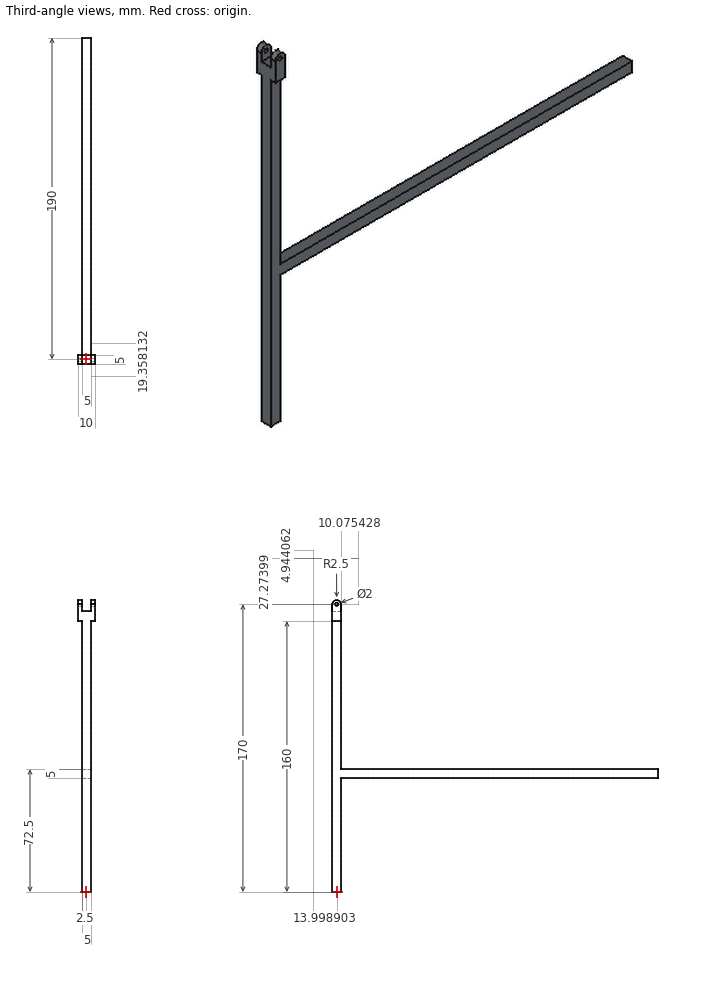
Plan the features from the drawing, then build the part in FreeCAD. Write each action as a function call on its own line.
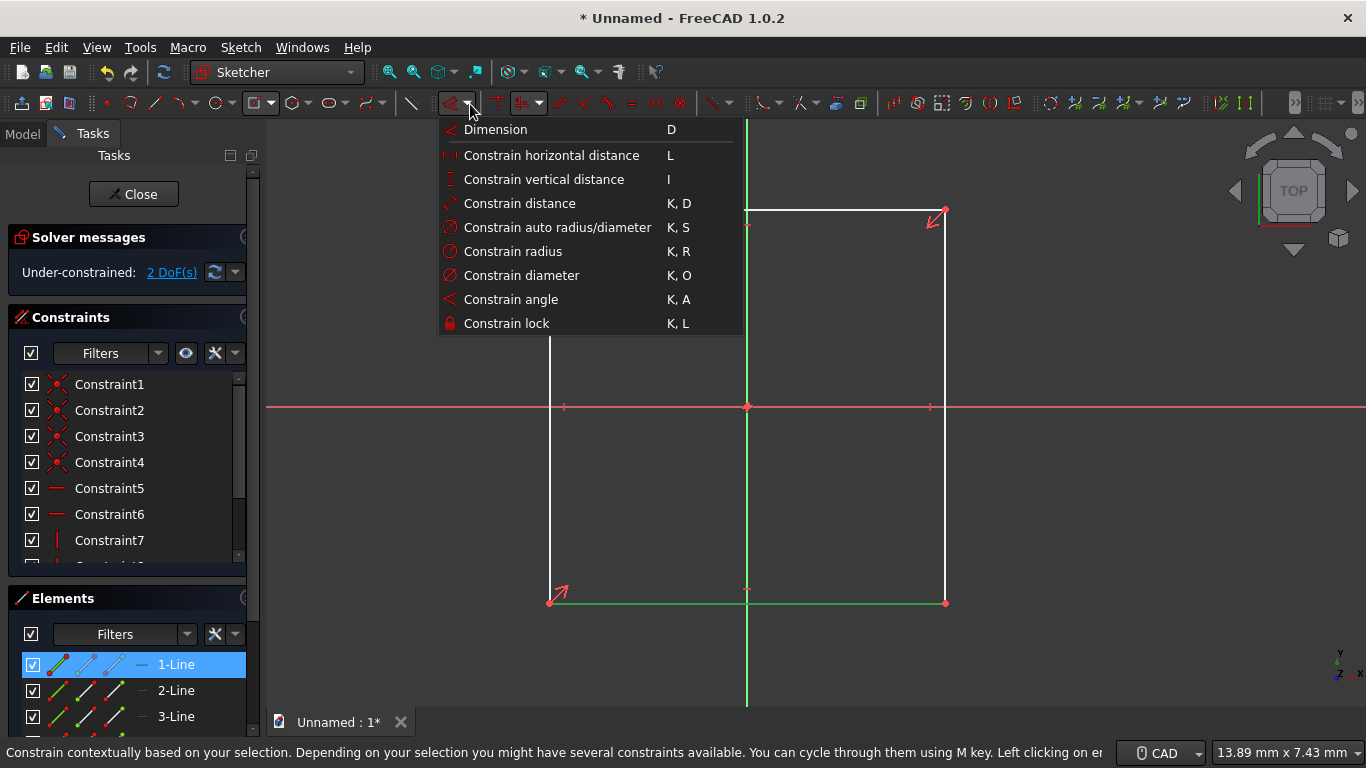
click(591, 155)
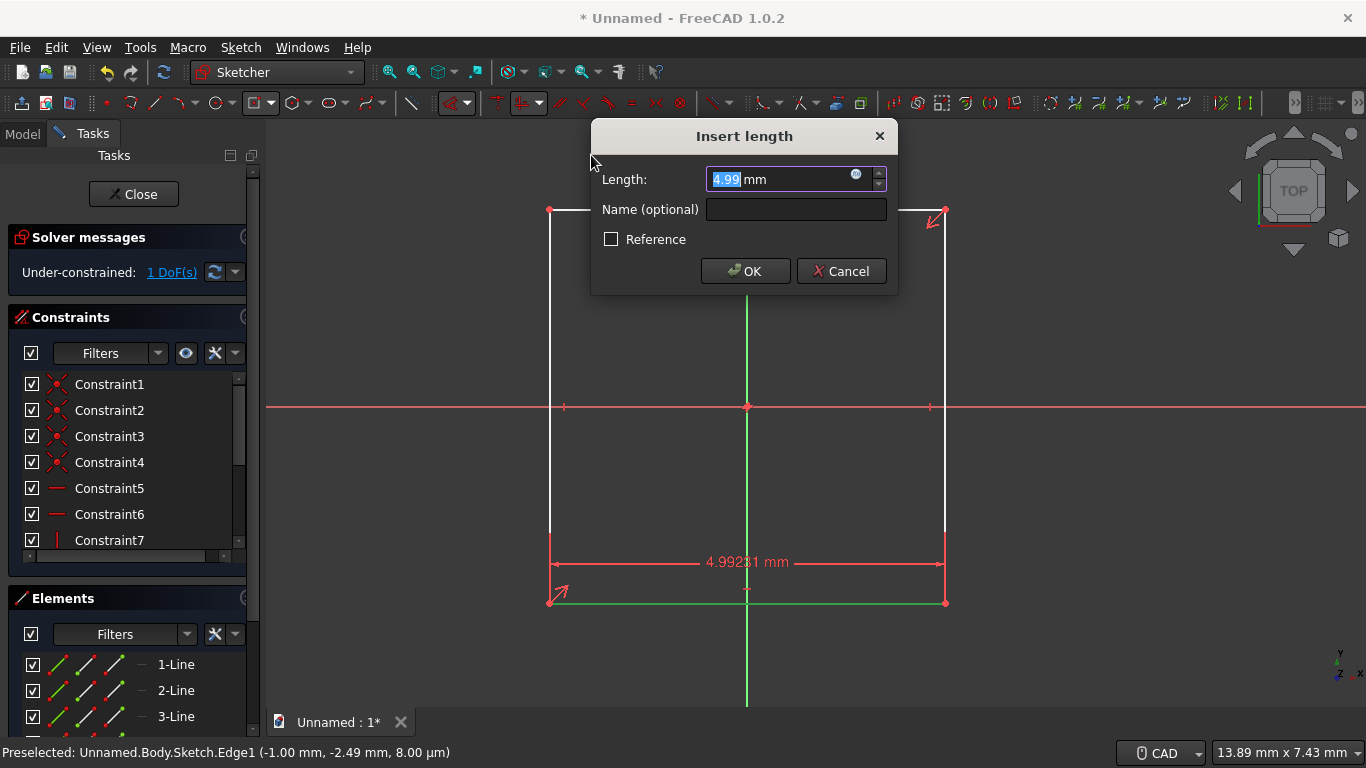
text(5)
key(Return)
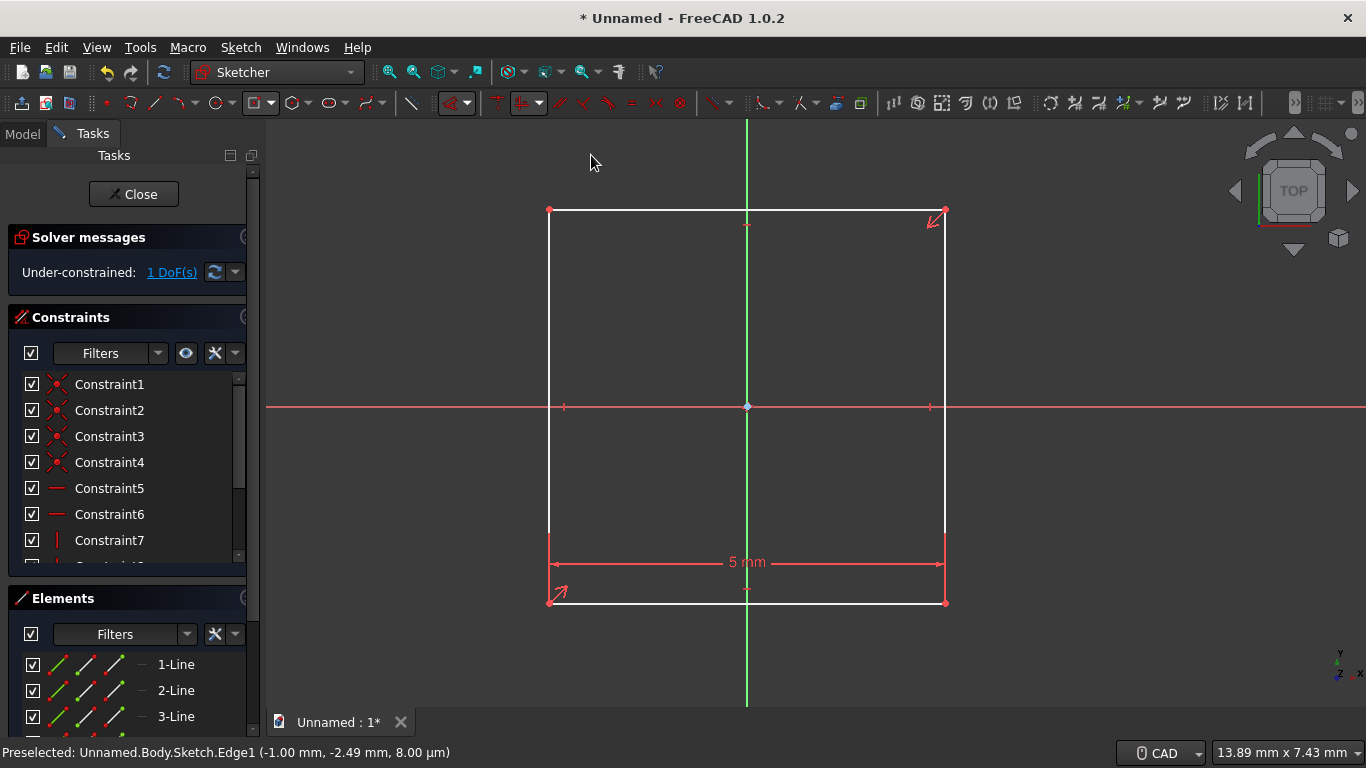
click(945, 485)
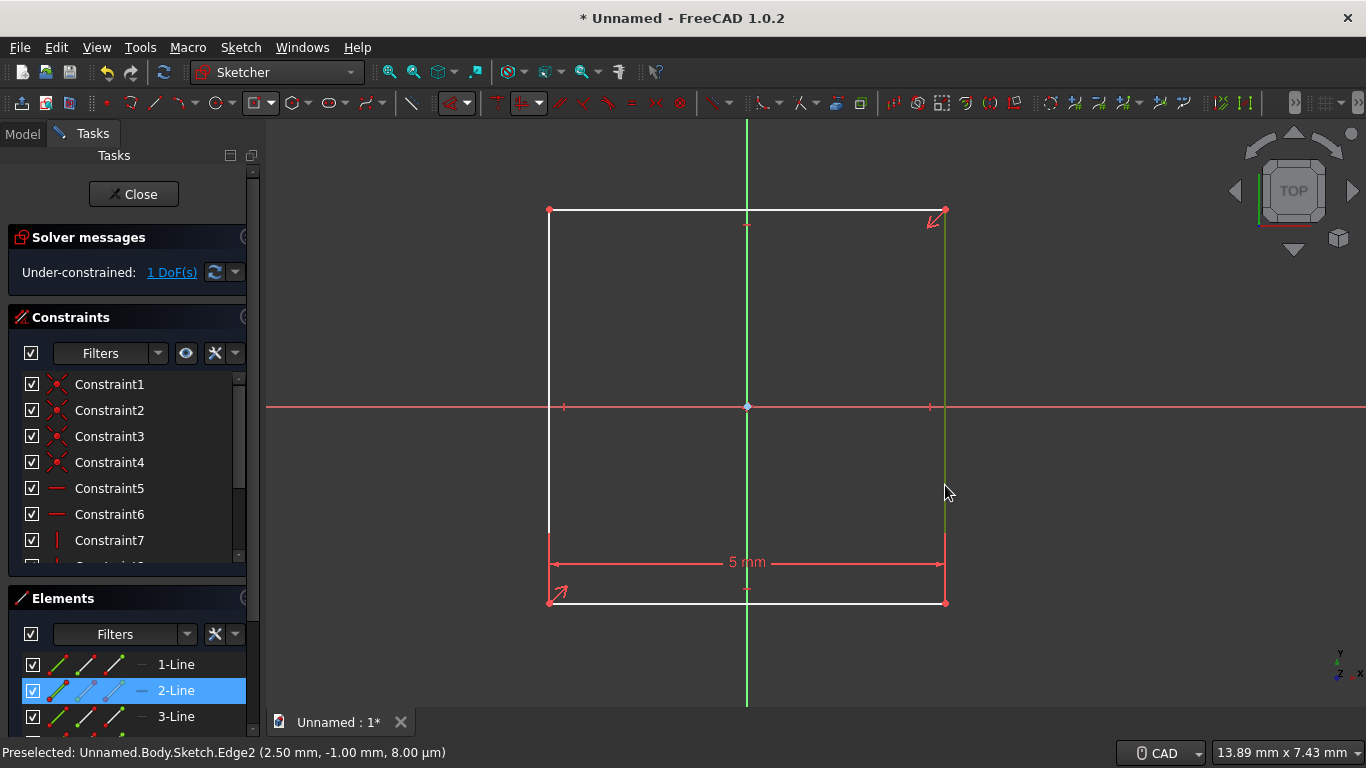
click(470, 104)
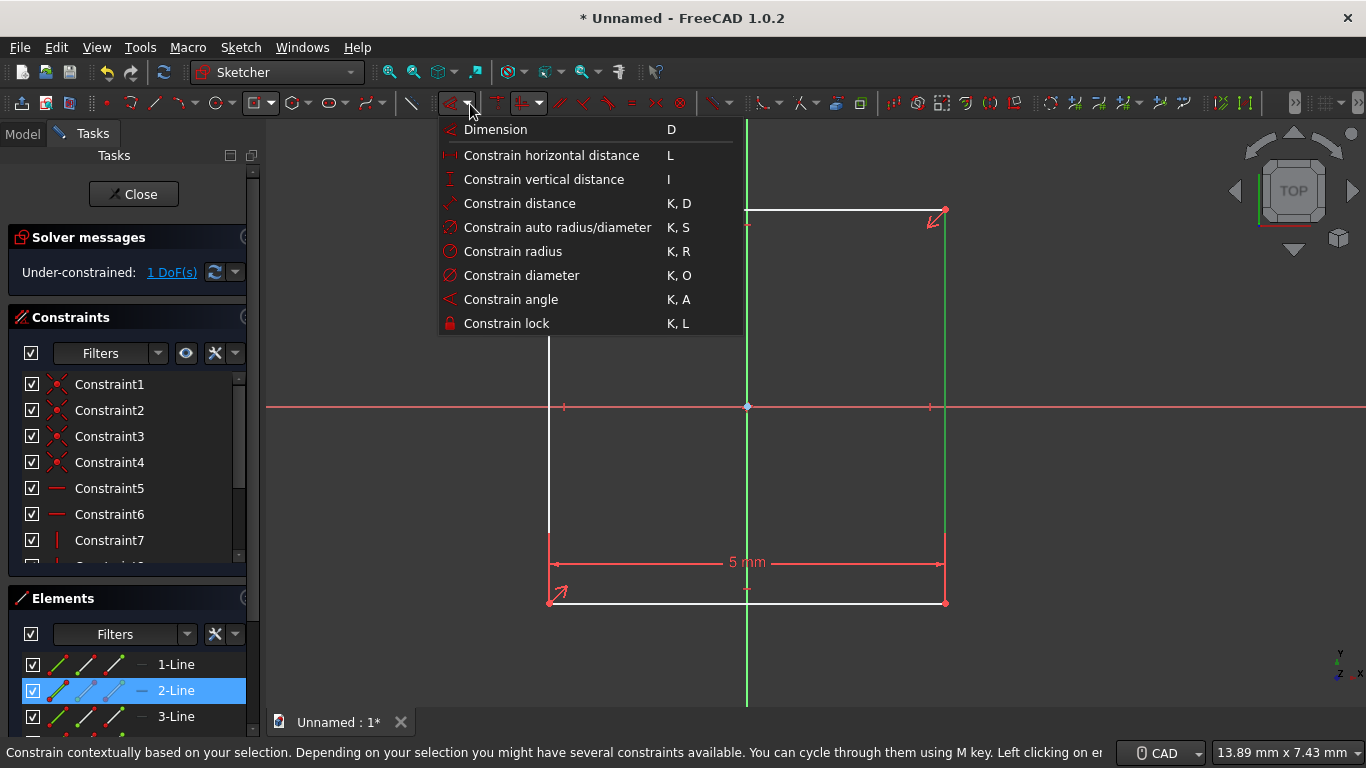
click(591, 179)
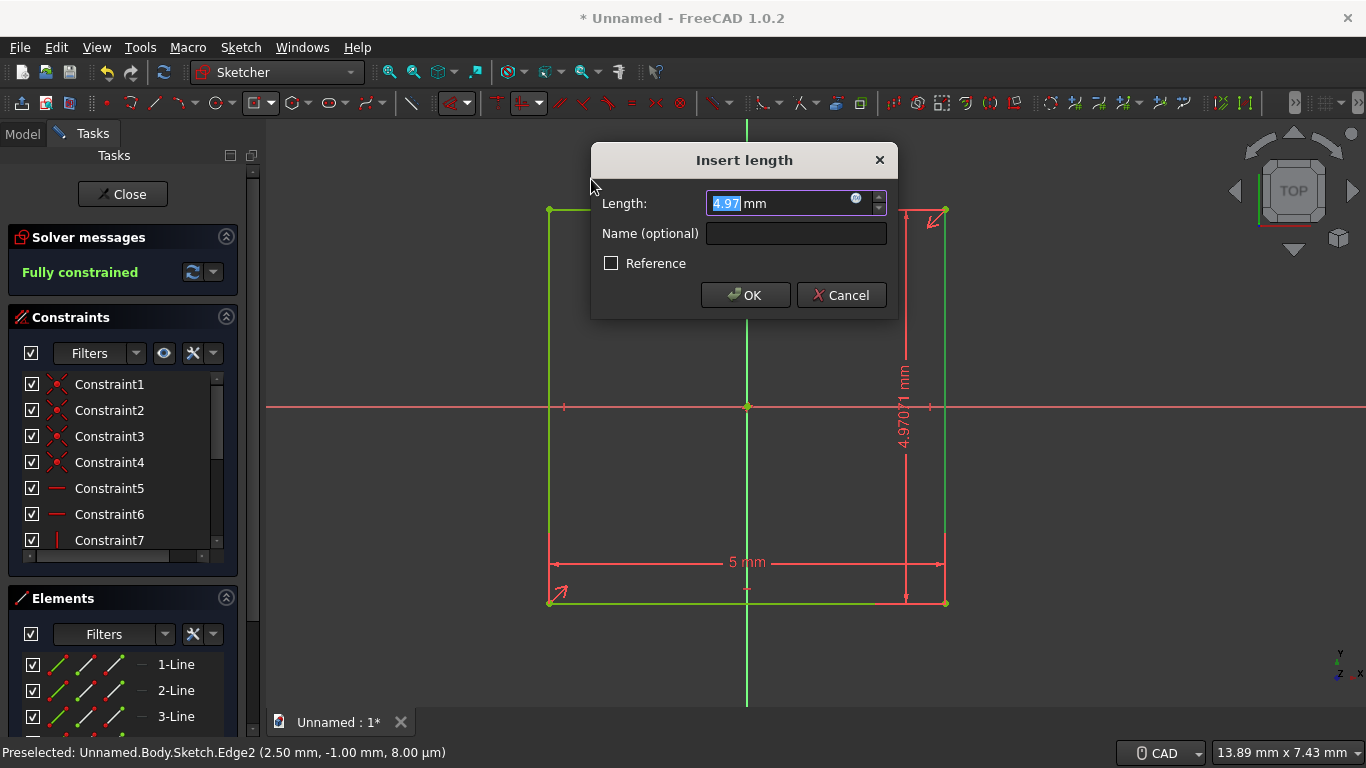
text(5)
key(Return)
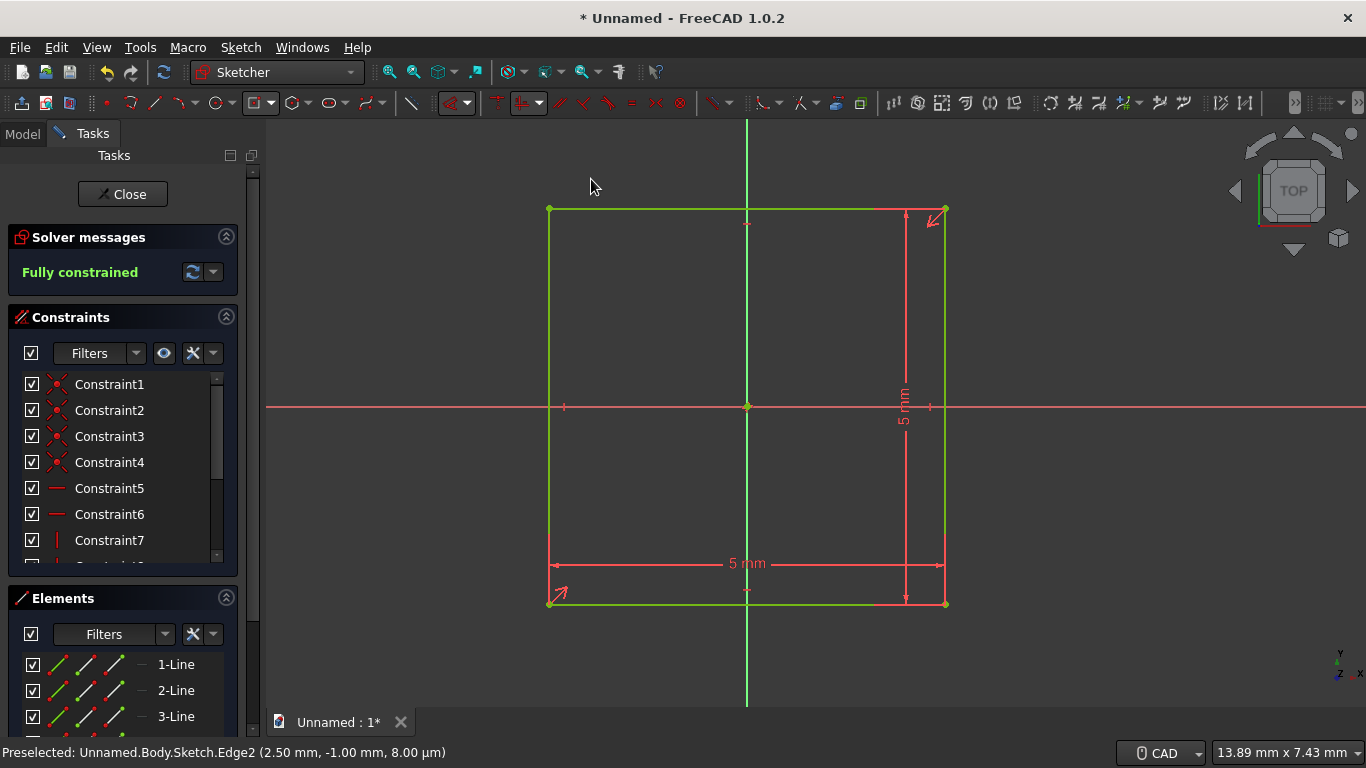
click(123, 194)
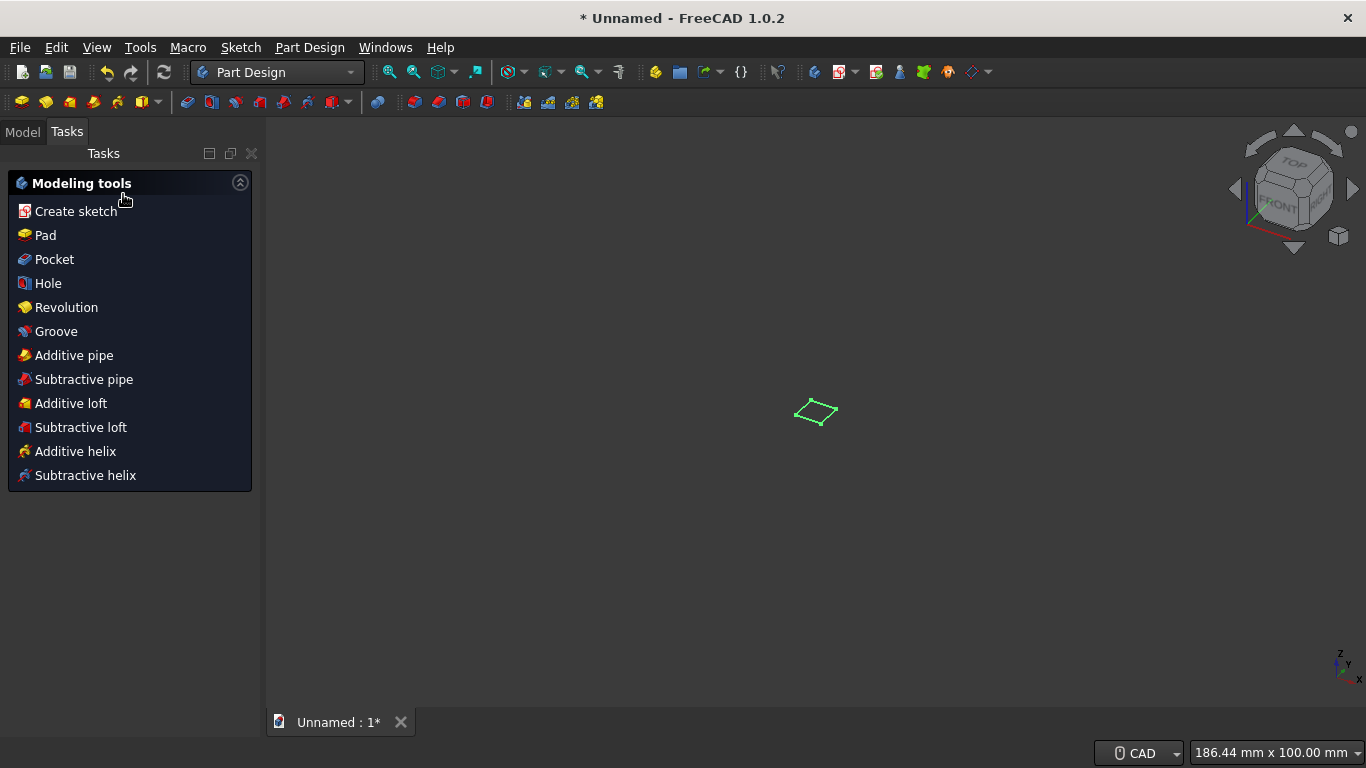
click(22, 102)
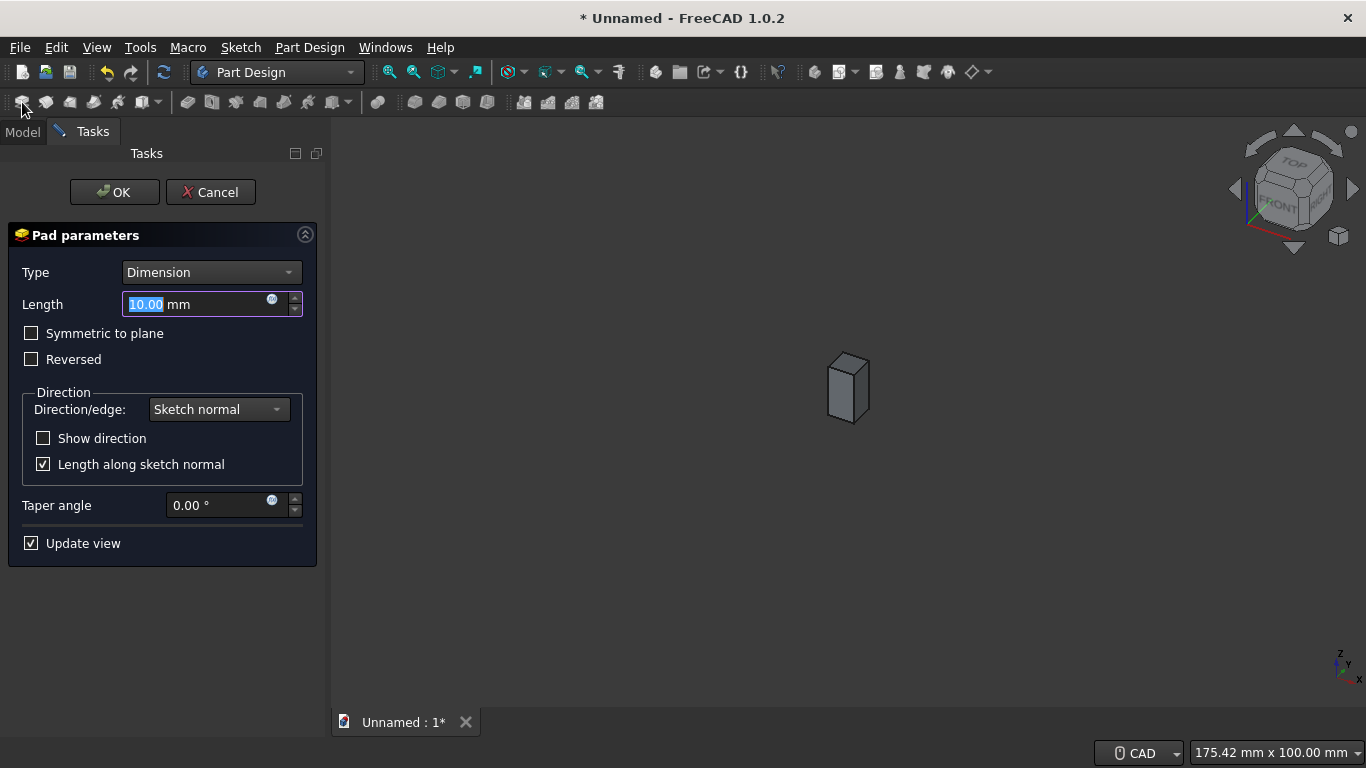
text(160)
key(Tab)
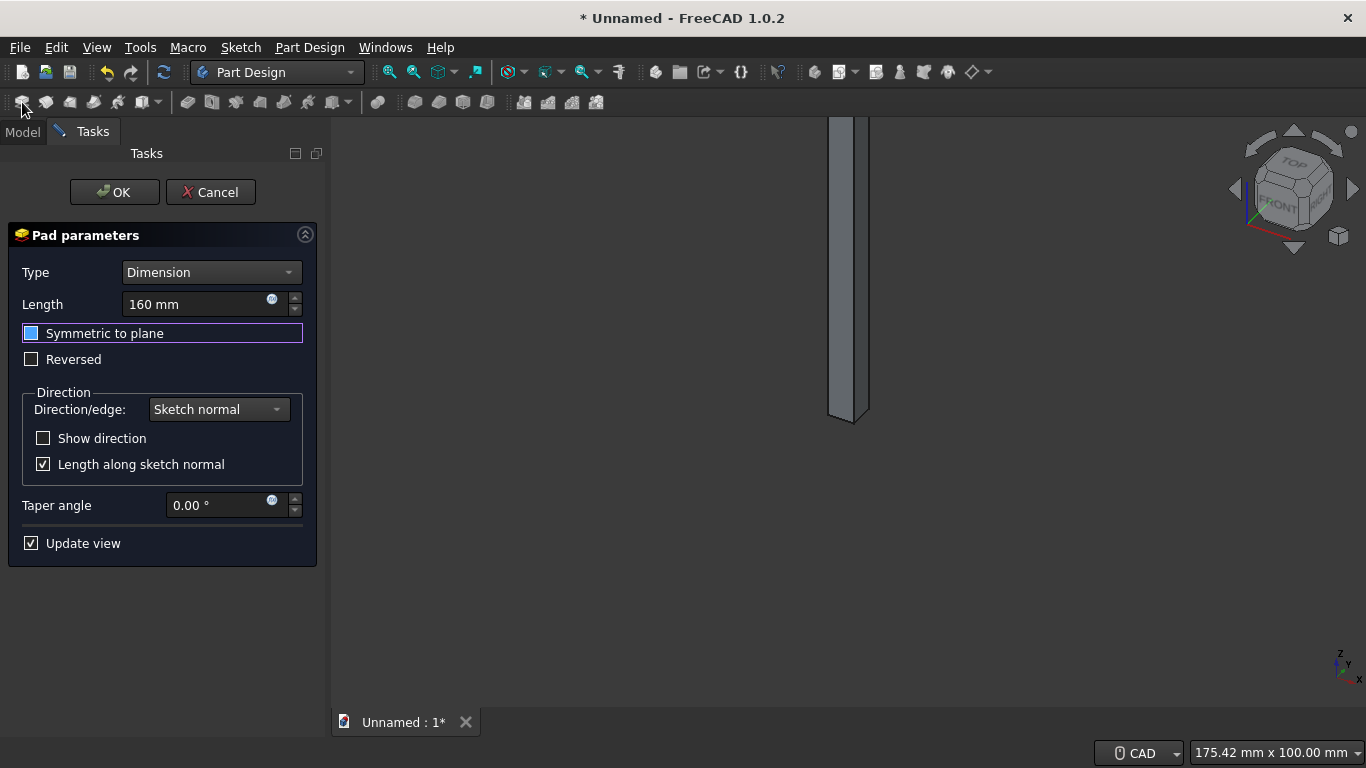
click(115, 192)